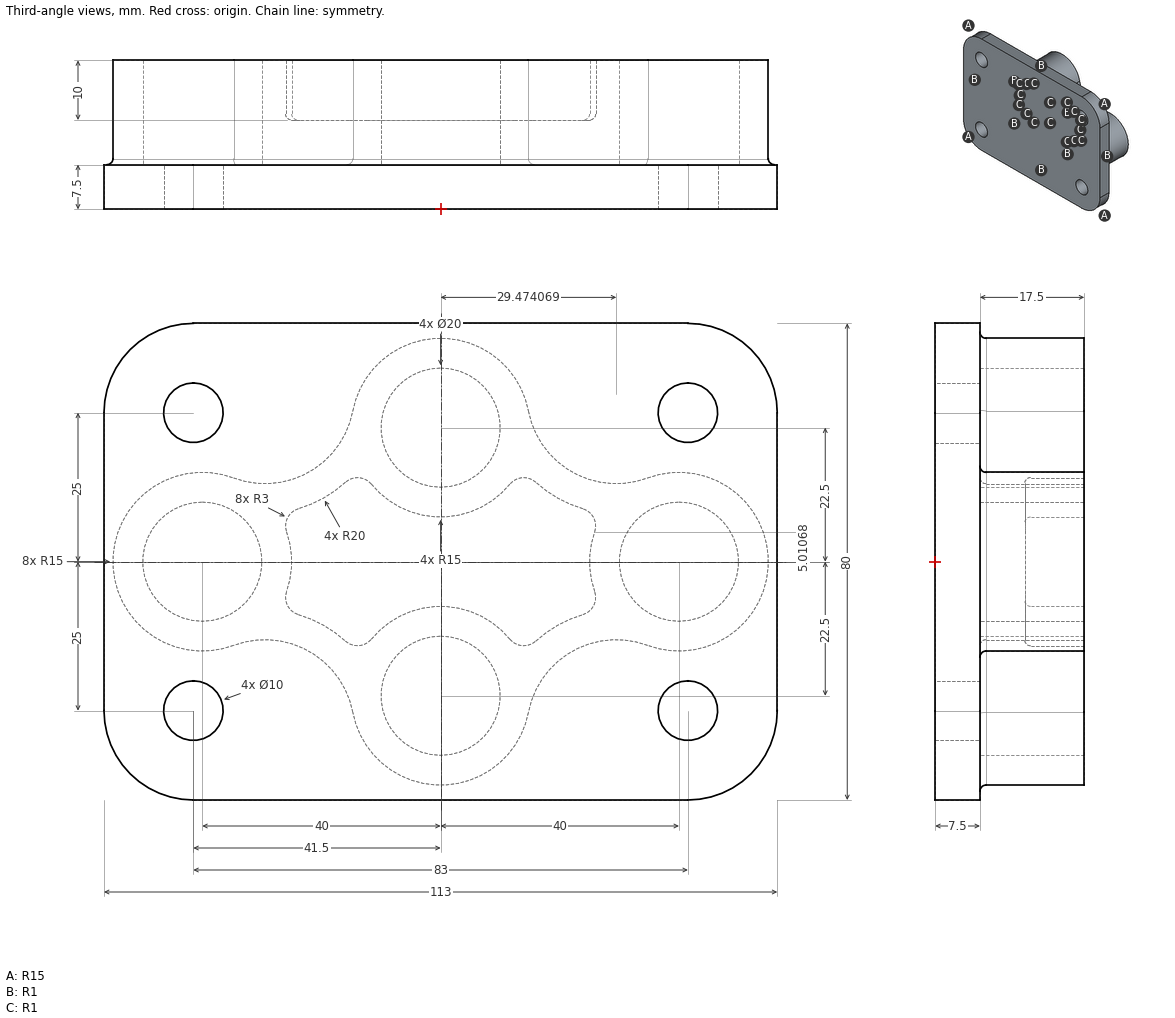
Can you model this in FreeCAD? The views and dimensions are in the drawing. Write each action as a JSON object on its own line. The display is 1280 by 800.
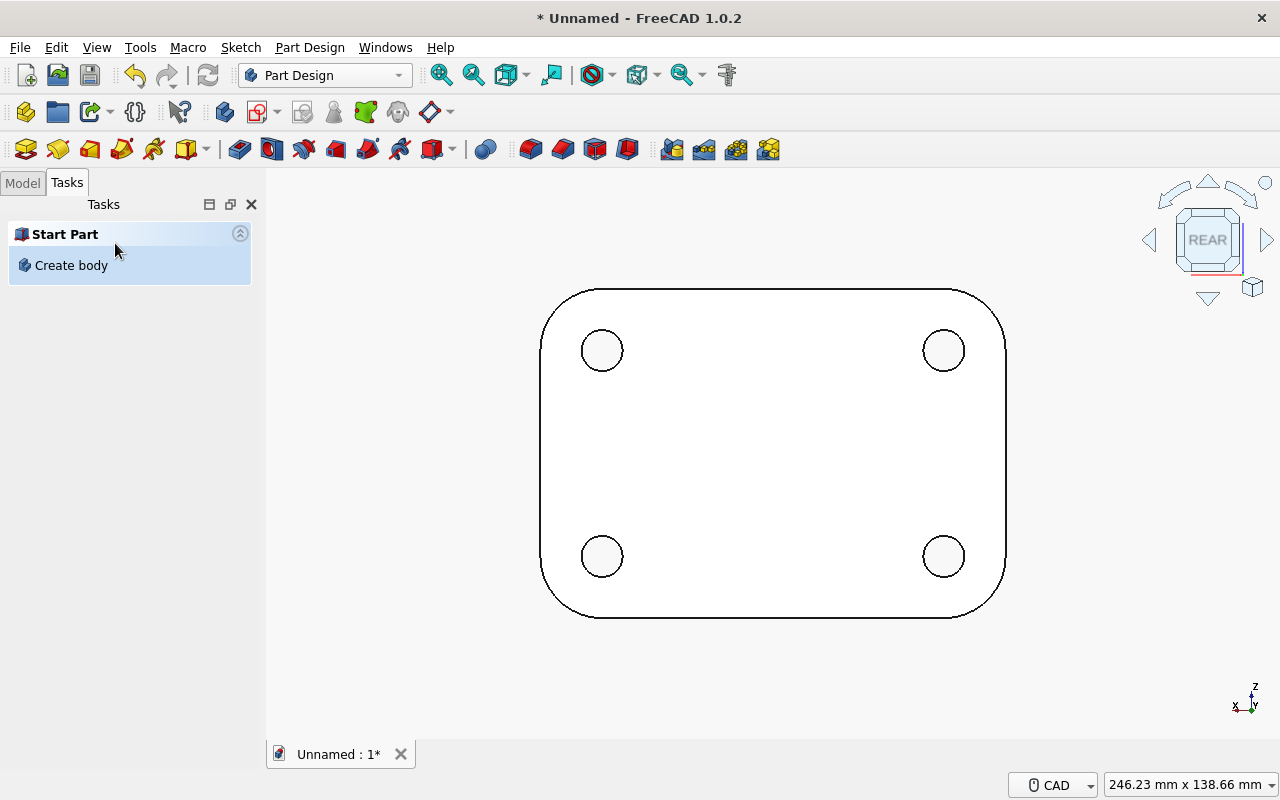
{"action": "left_click", "coordinate": [773, 452]}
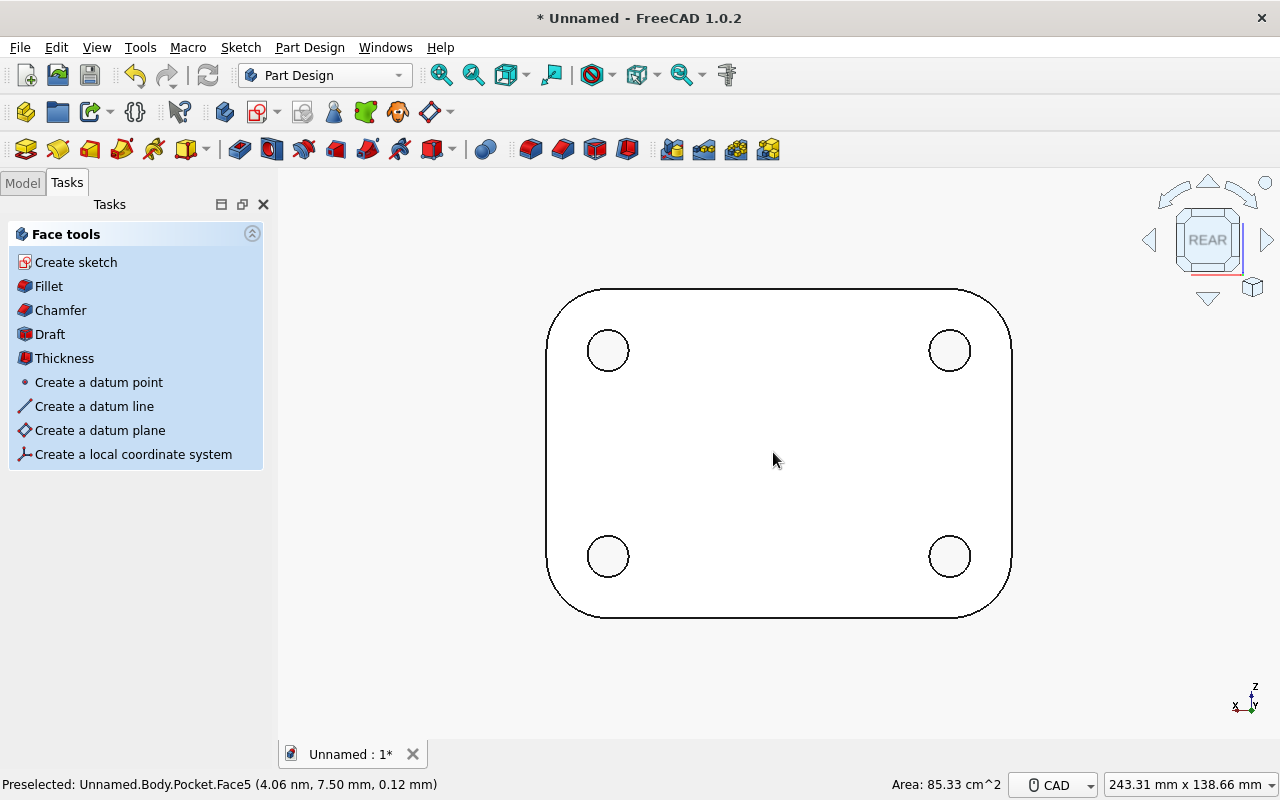
{"action": "left_click", "coordinate": [258, 112]}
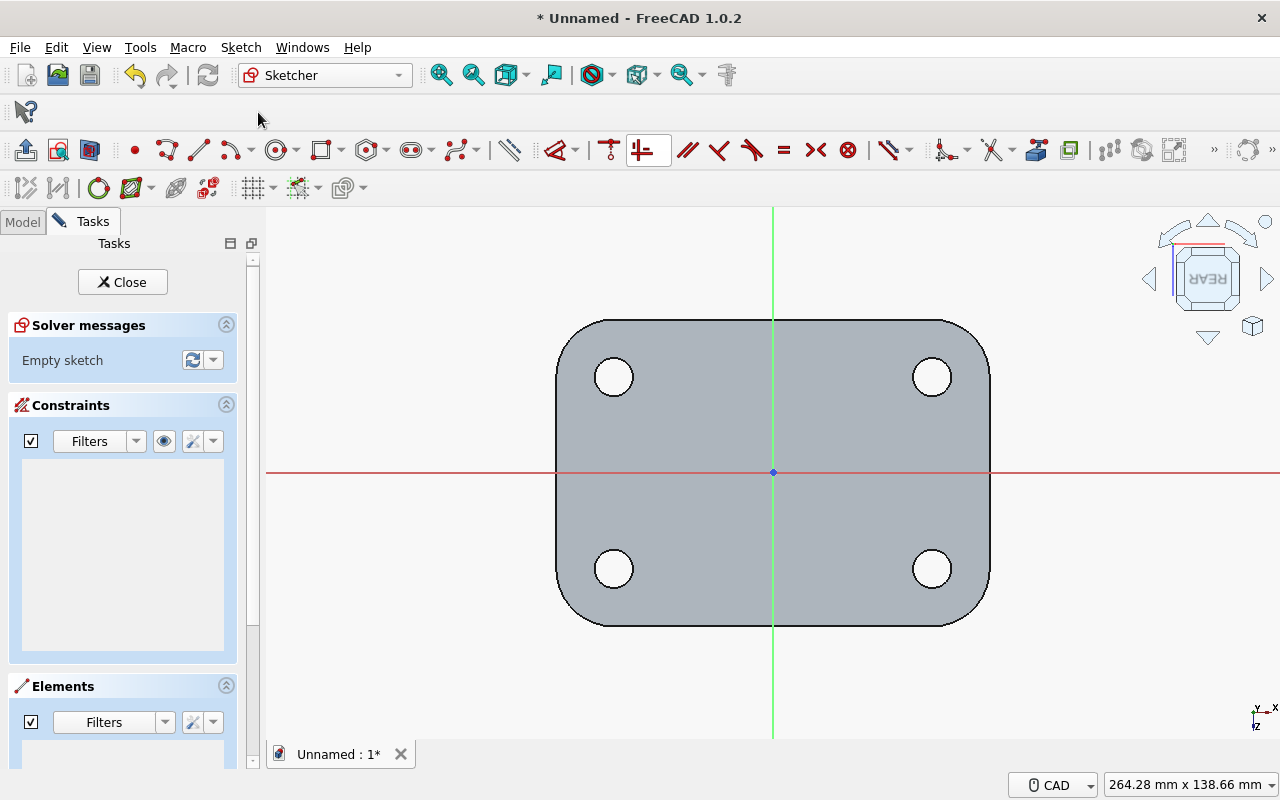
{"action": "key", "text": "g 3 a"}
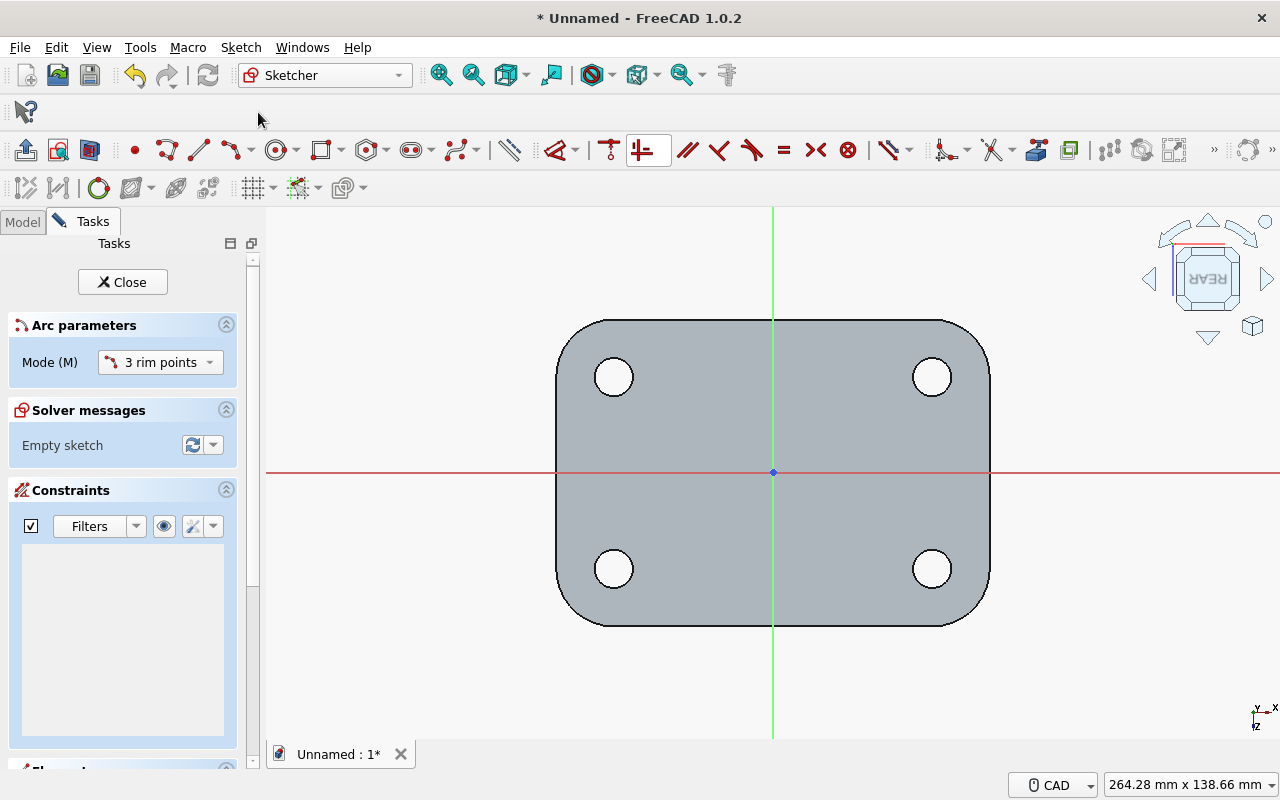
{"action": "left_click", "coordinate": [716, 570]}
{"action": "left_click", "coordinate": [830, 570]}
{"action": "left_click", "coordinate": [757, 615]}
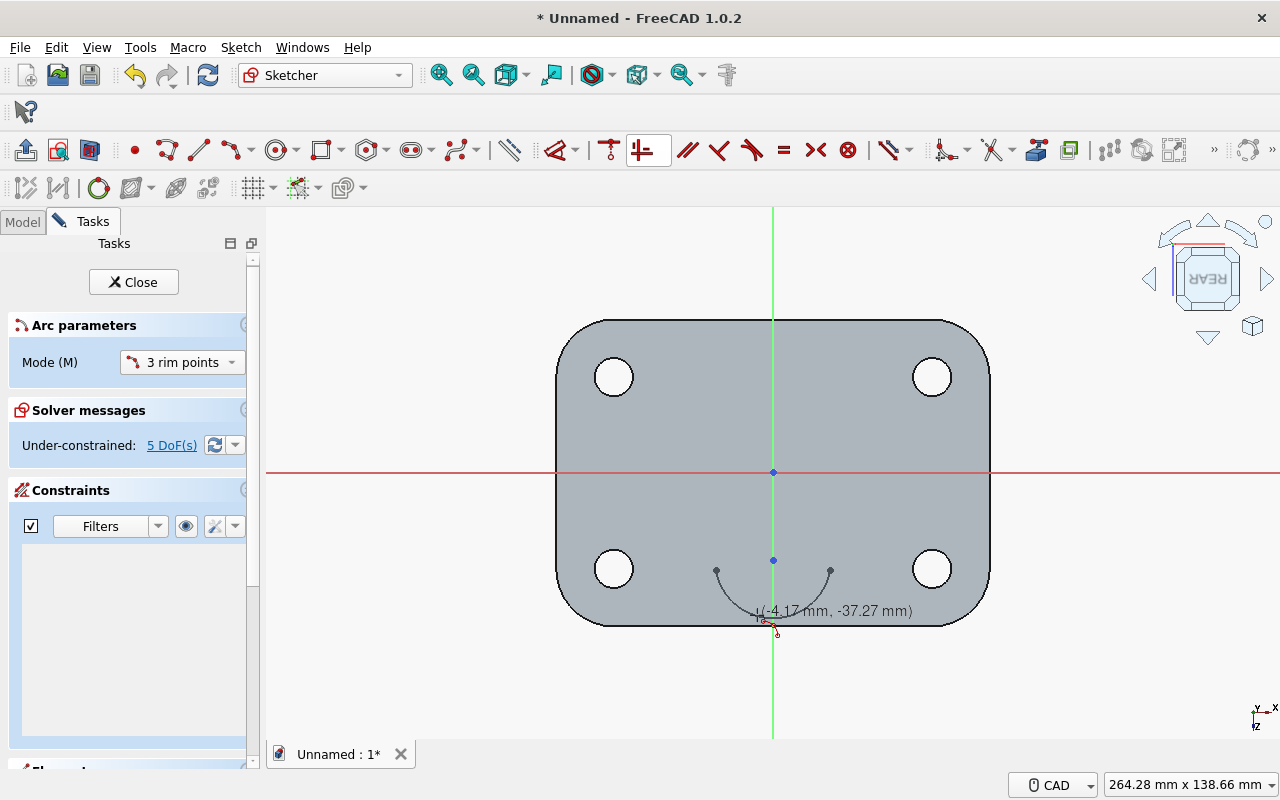
{"action": "left_click", "coordinate": [830, 571]}
{"action": "left_click", "coordinate": [906, 527]}
{"action": "left_click", "coordinate": [858, 531]}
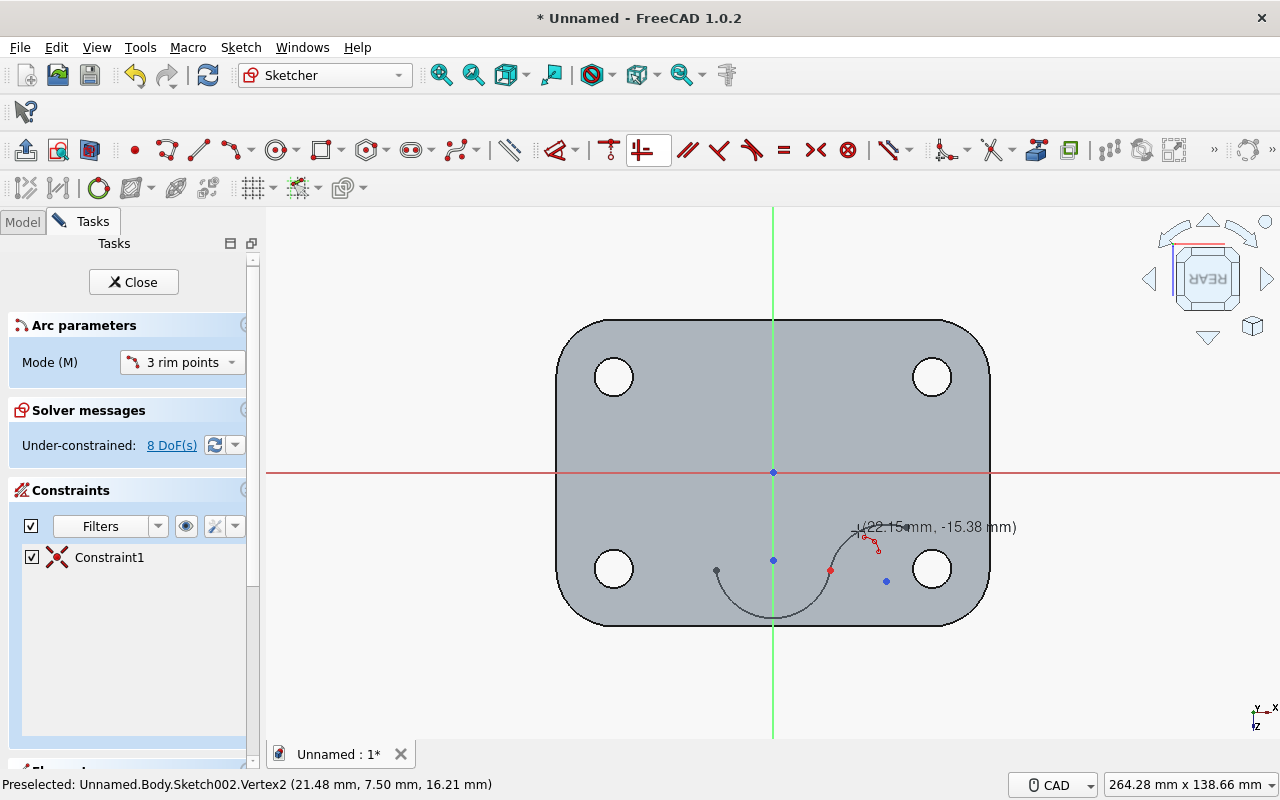
{"action": "left_click", "coordinate": [906, 528]}
{"action": "left_click", "coordinate": [906, 419]}
{"action": "left_click", "coordinate": [980, 495]}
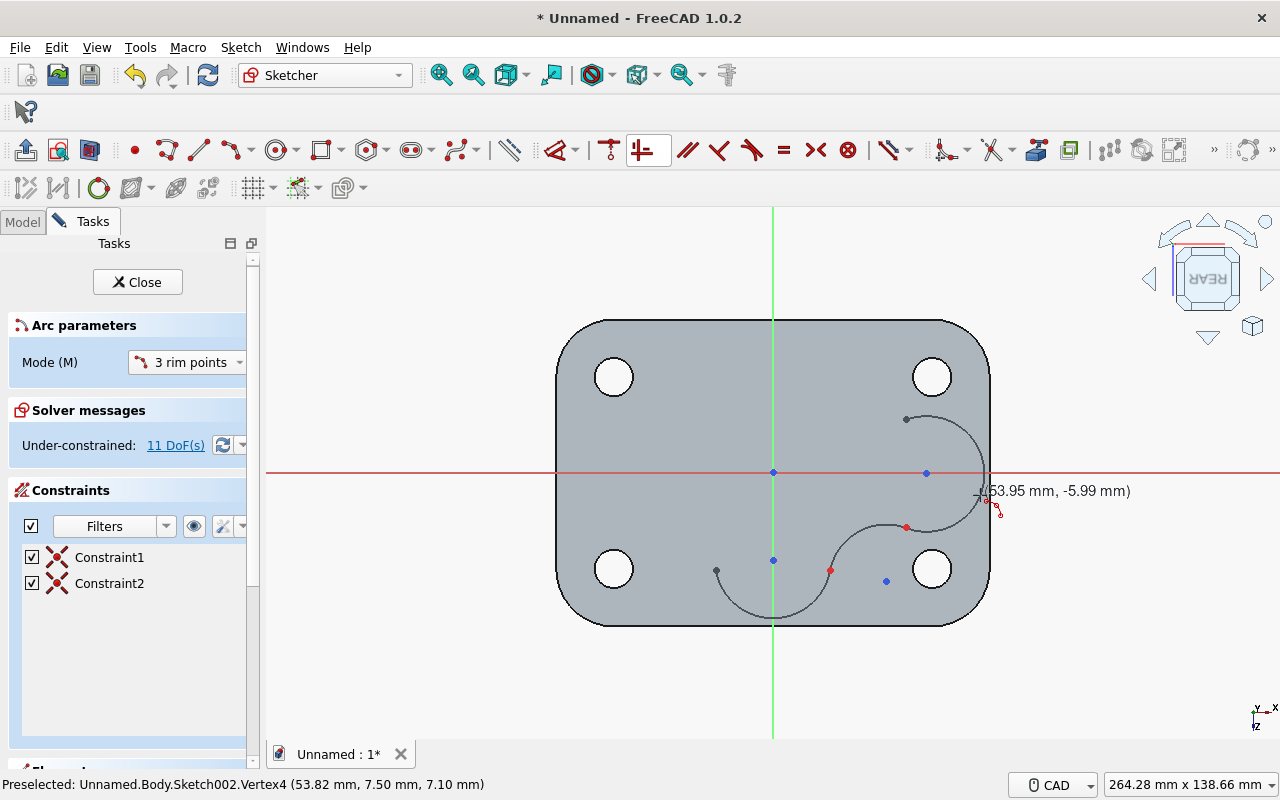
{"action": "left_click", "coordinate": [906, 420]}
{"action": "left_click", "coordinate": [830, 376]}
{"action": "left_click", "coordinate": [858, 415]}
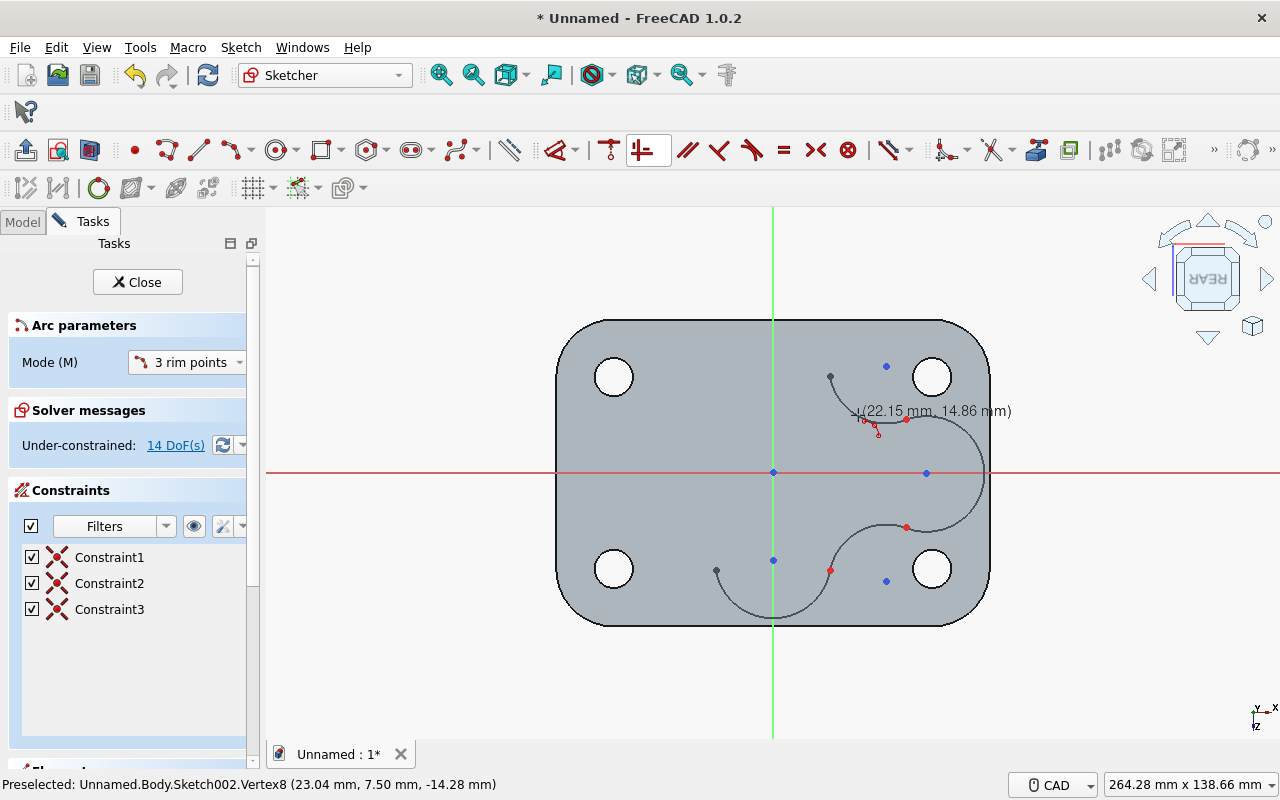
{"action": "left_click", "coordinate": [830, 377]}
{"action": "left_click", "coordinate": [716, 376]}
{"action": "left_click", "coordinate": [789, 331]}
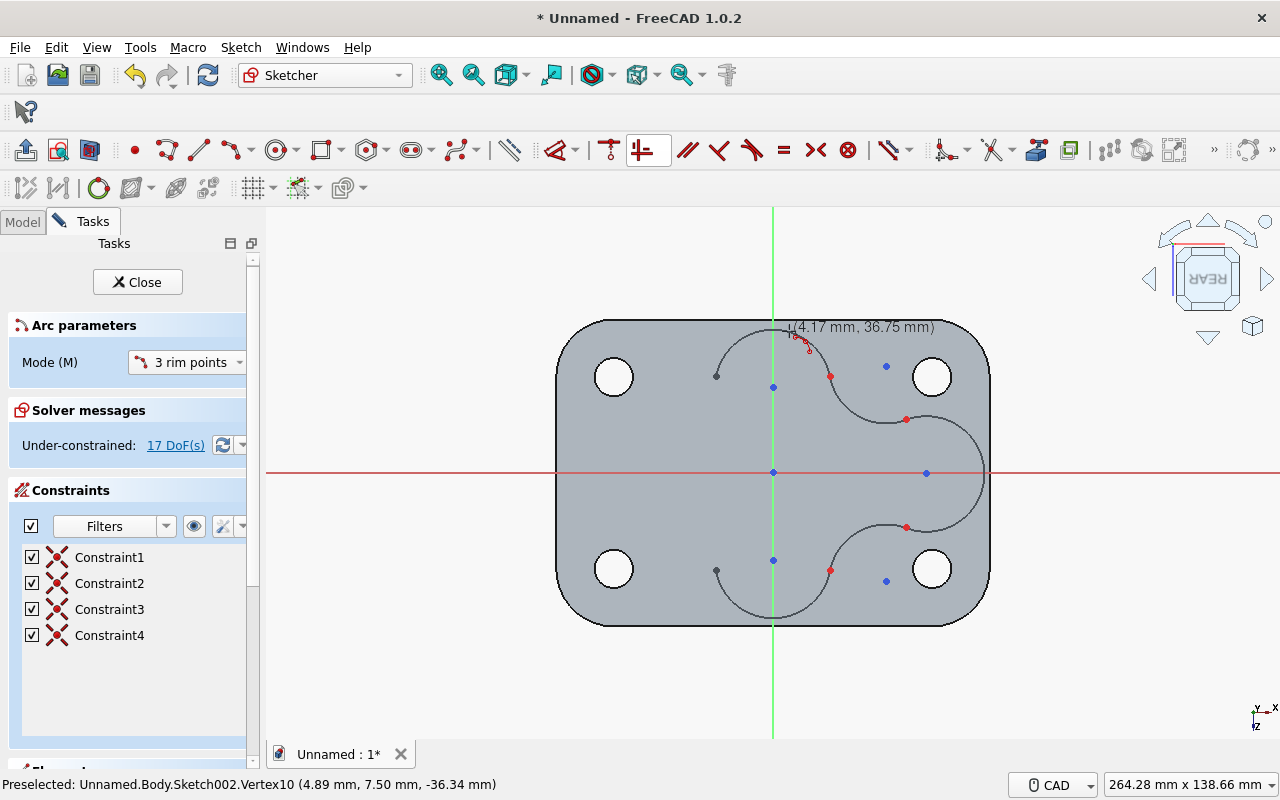
{"action": "left_click", "coordinate": [716, 377]}
{"action": "left_click", "coordinate": [640, 419]}
{"action": "left_click", "coordinate": [688, 415]}